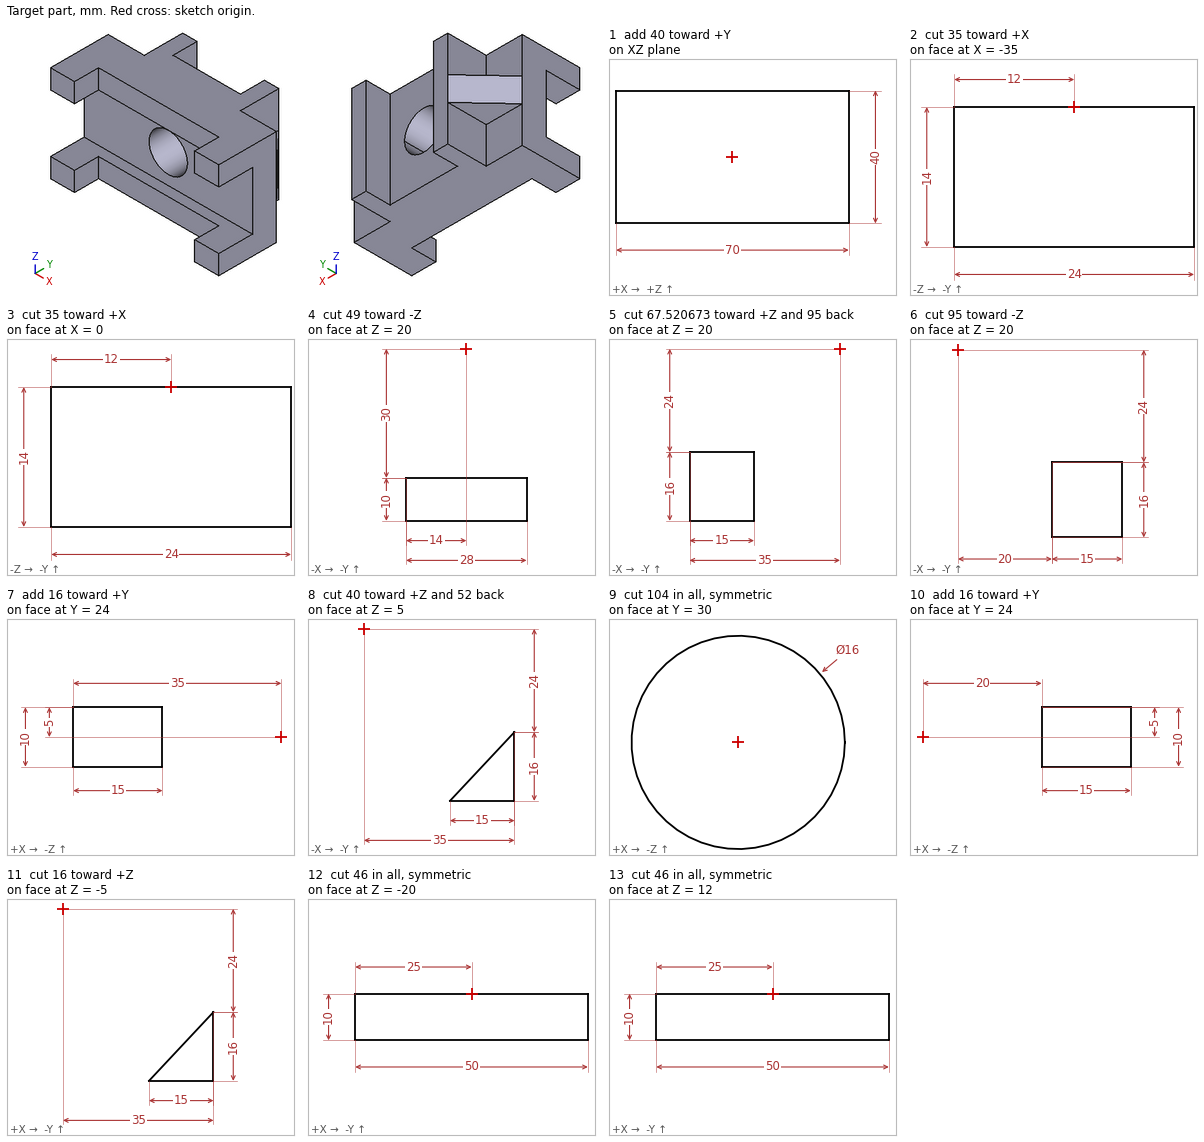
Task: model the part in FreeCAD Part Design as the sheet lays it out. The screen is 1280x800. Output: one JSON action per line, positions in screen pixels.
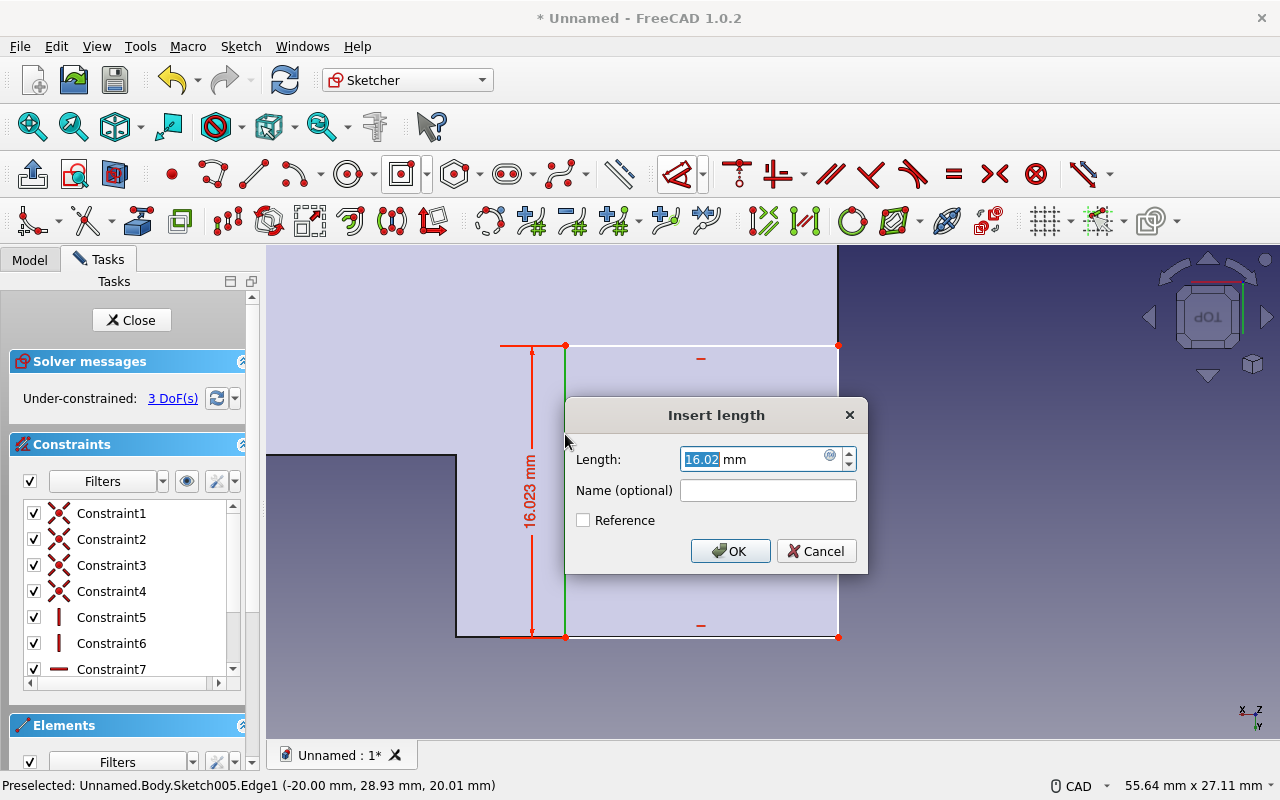
{"action": "type", "text": "16"}
{"action": "key", "text": "Return"}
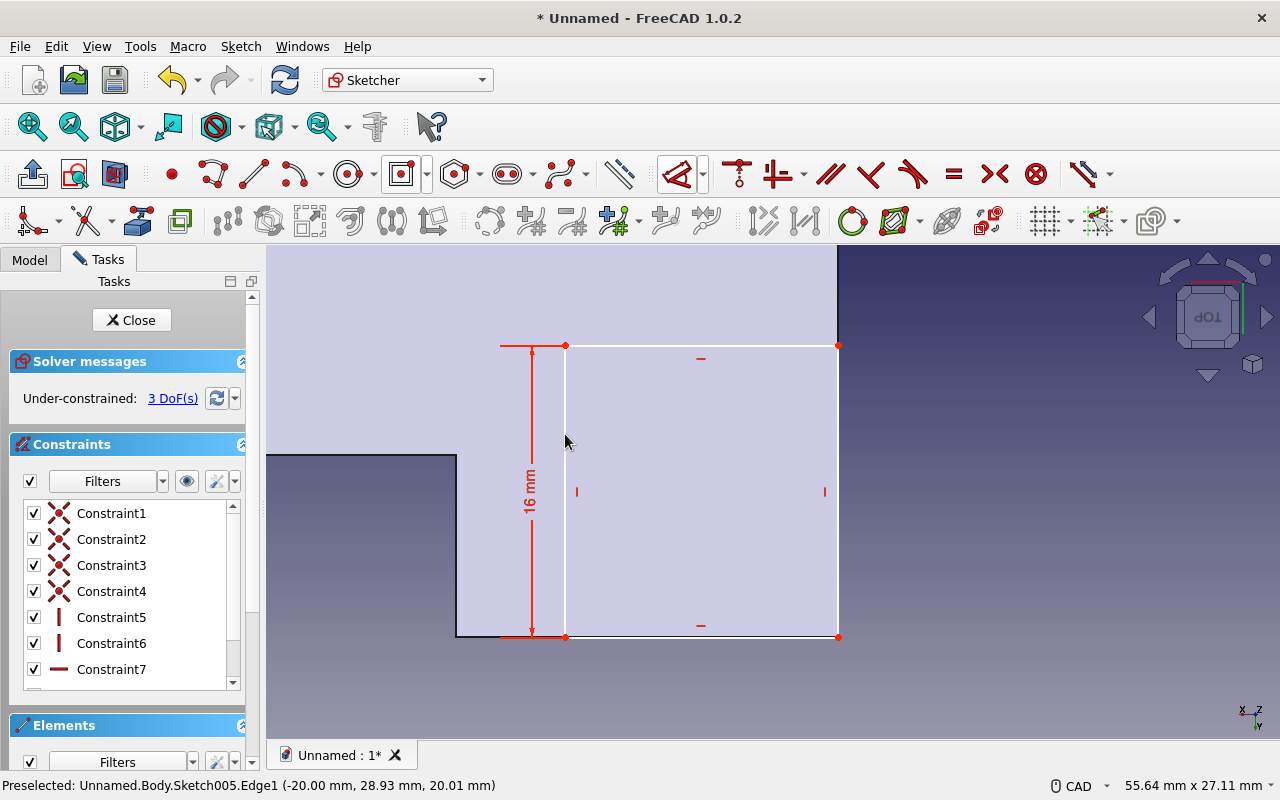
{"action": "left_click", "coordinate": [647, 638]}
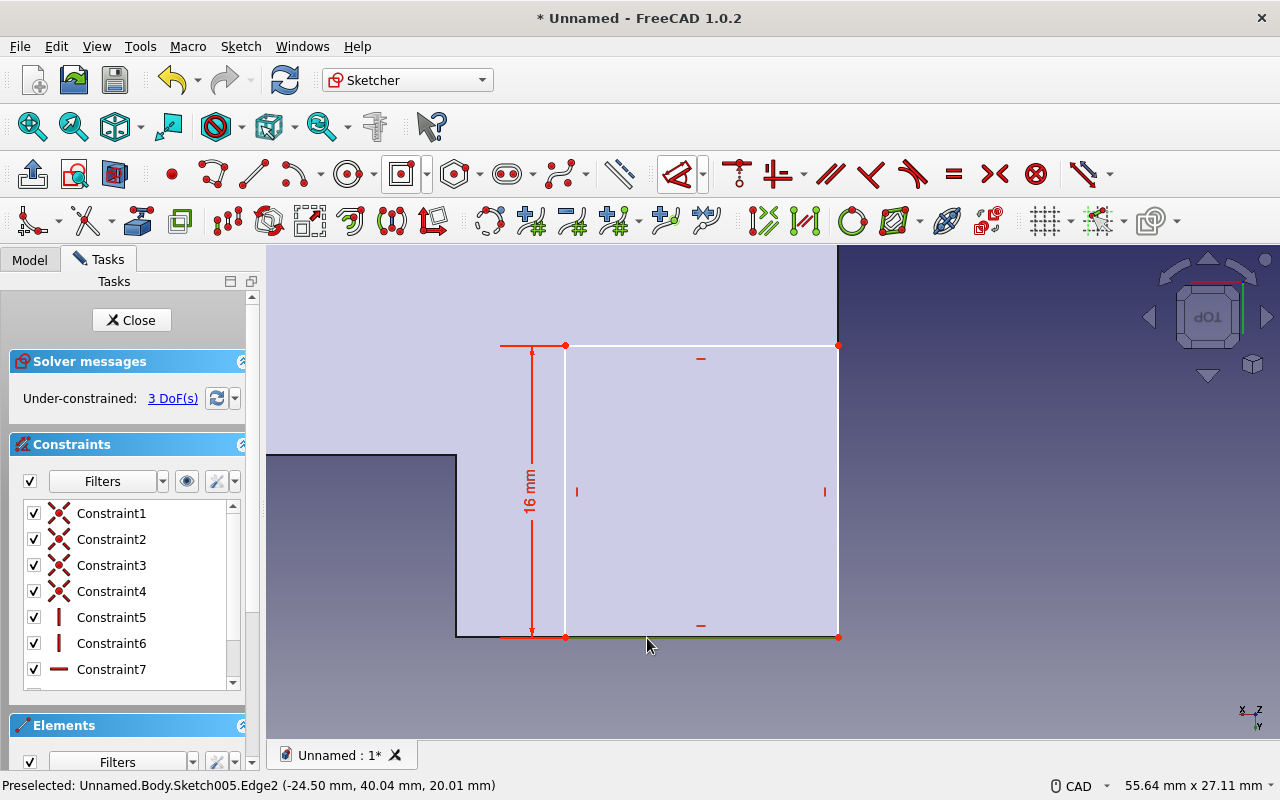
{"action": "key", "text": "l"}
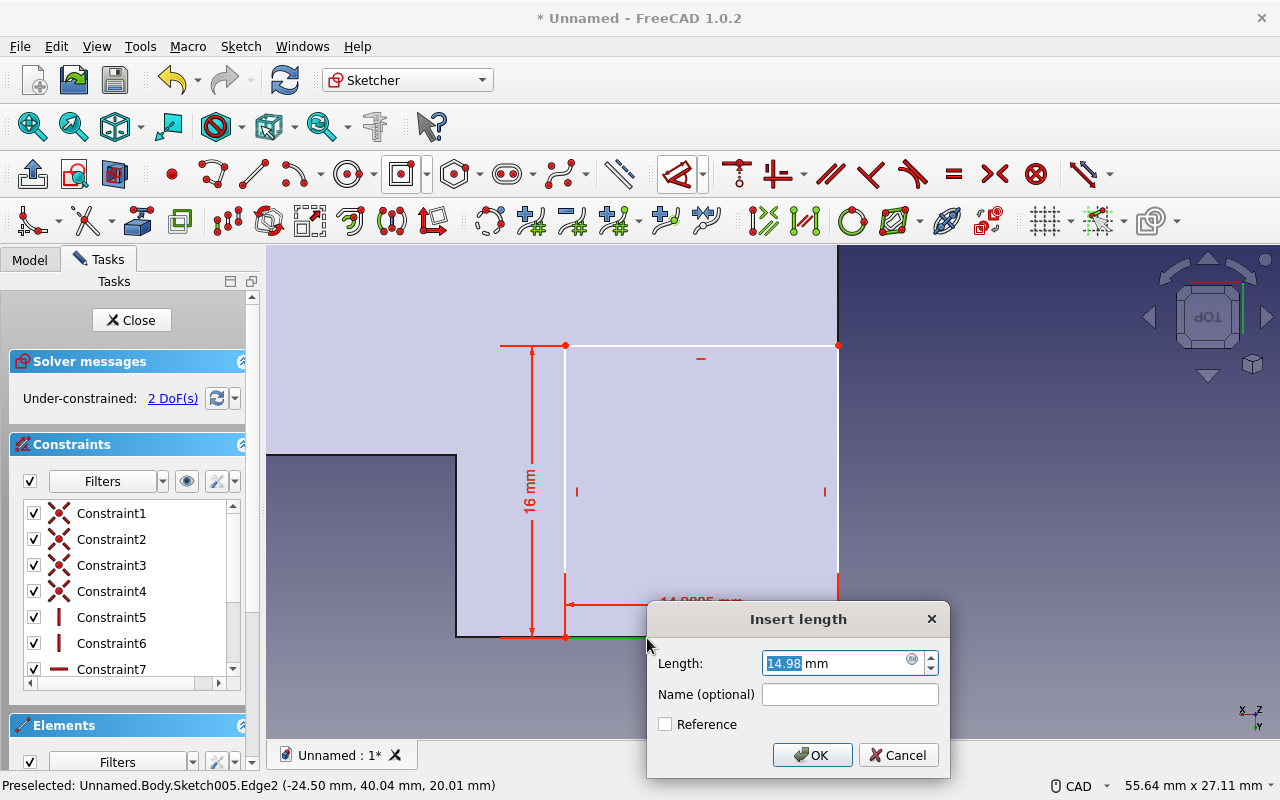
{"action": "type", "text": "15"}
{"action": "key", "text": "Return"}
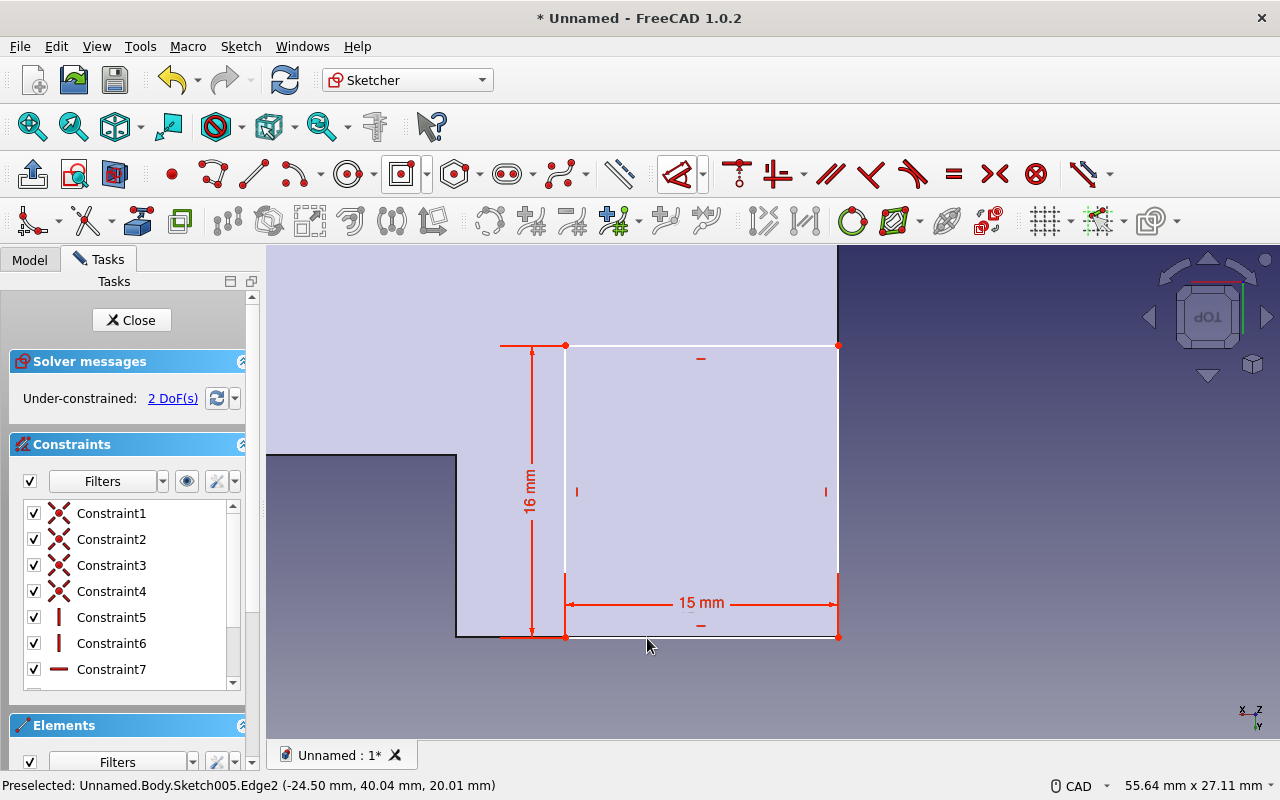
{"action": "left_click", "coordinate": [565, 346]}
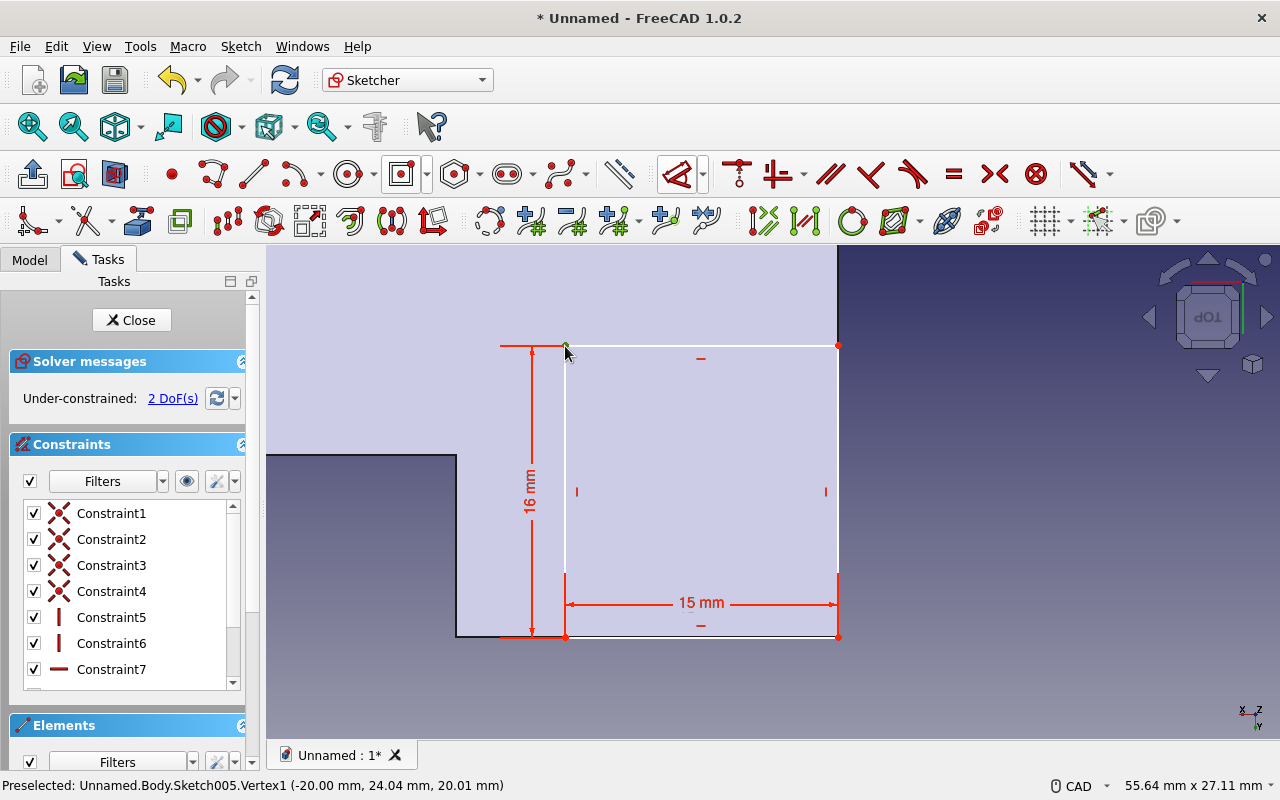
{"action": "key", "text": "l"}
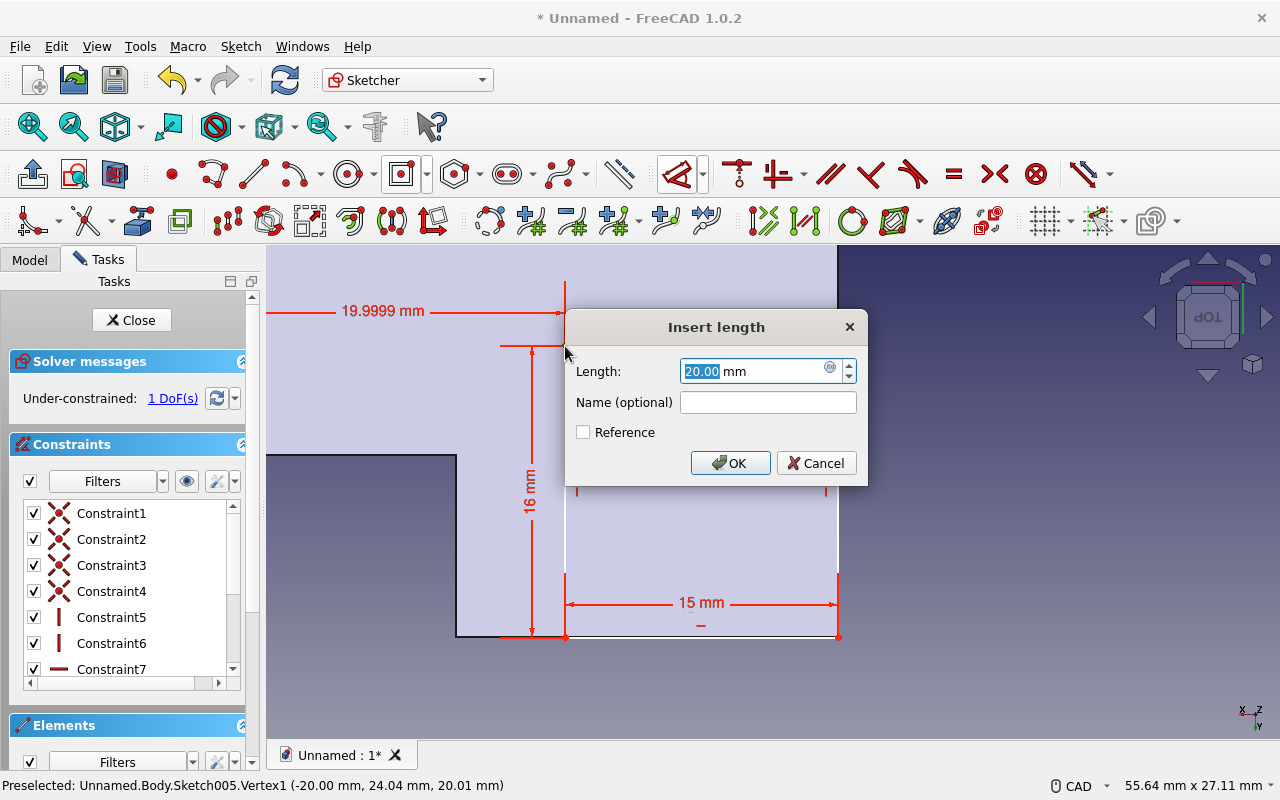
{"action": "type", "text": "20"}
{"action": "key", "text": "Return"}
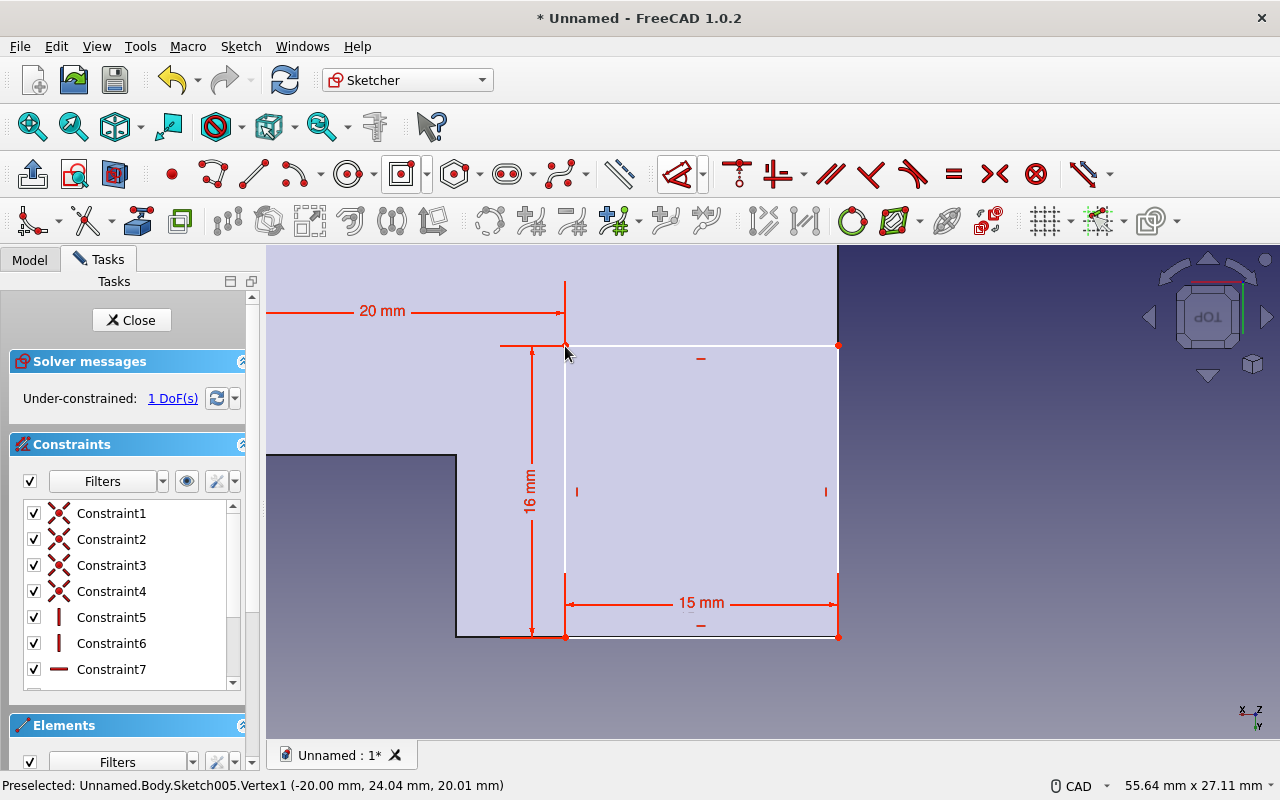
{"action": "left_click", "coordinate": [565, 346]}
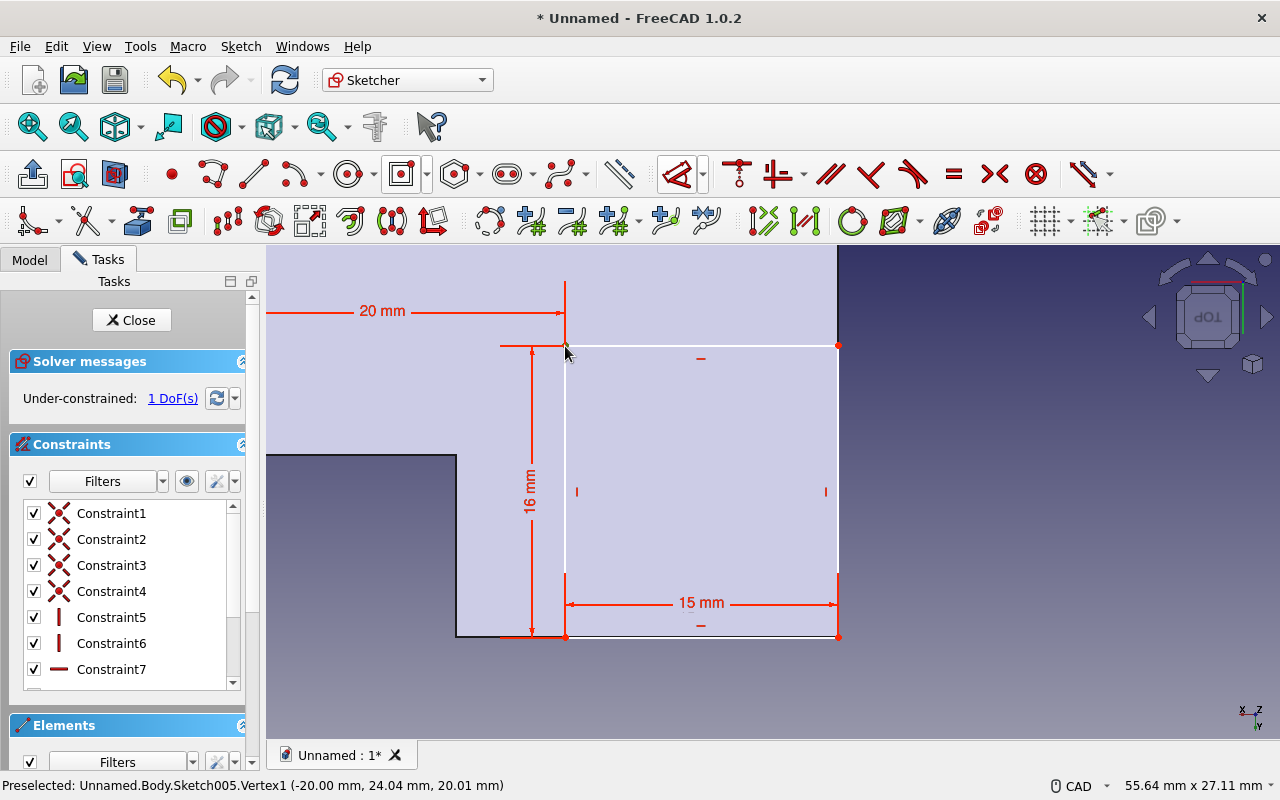
{"action": "left_click", "coordinate": [702, 174]}